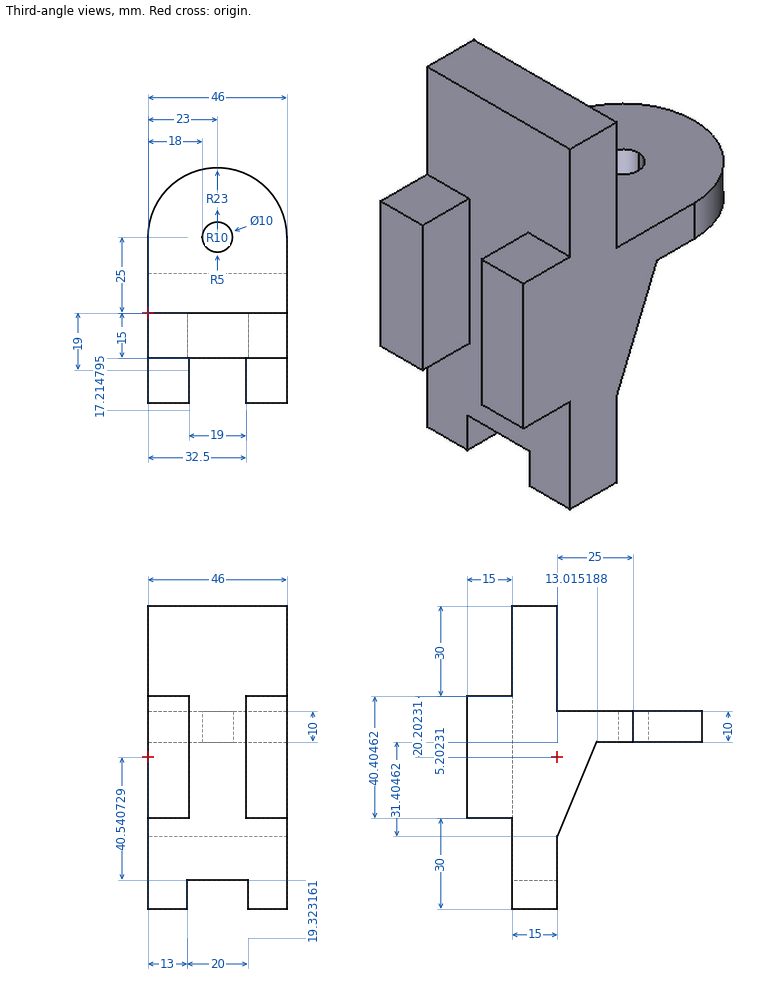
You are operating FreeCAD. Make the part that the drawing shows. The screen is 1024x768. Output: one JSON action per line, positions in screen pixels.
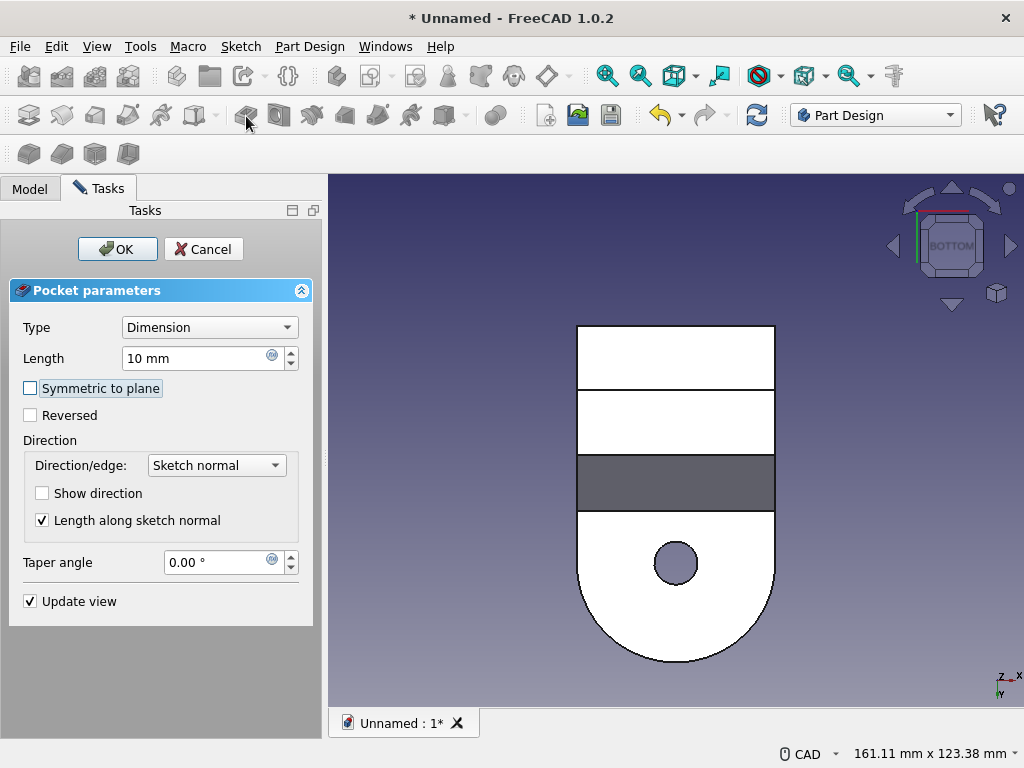
{"action": "left_click", "coordinate": [118, 249]}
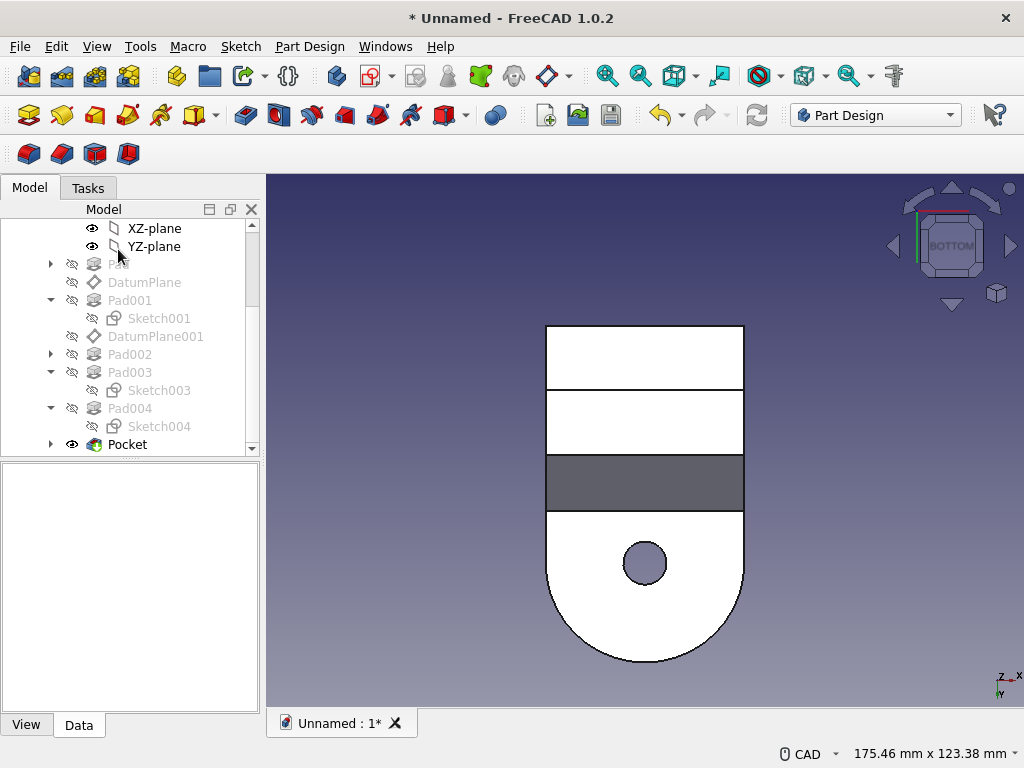
{"action": "left_click", "coordinate": [370, 76]}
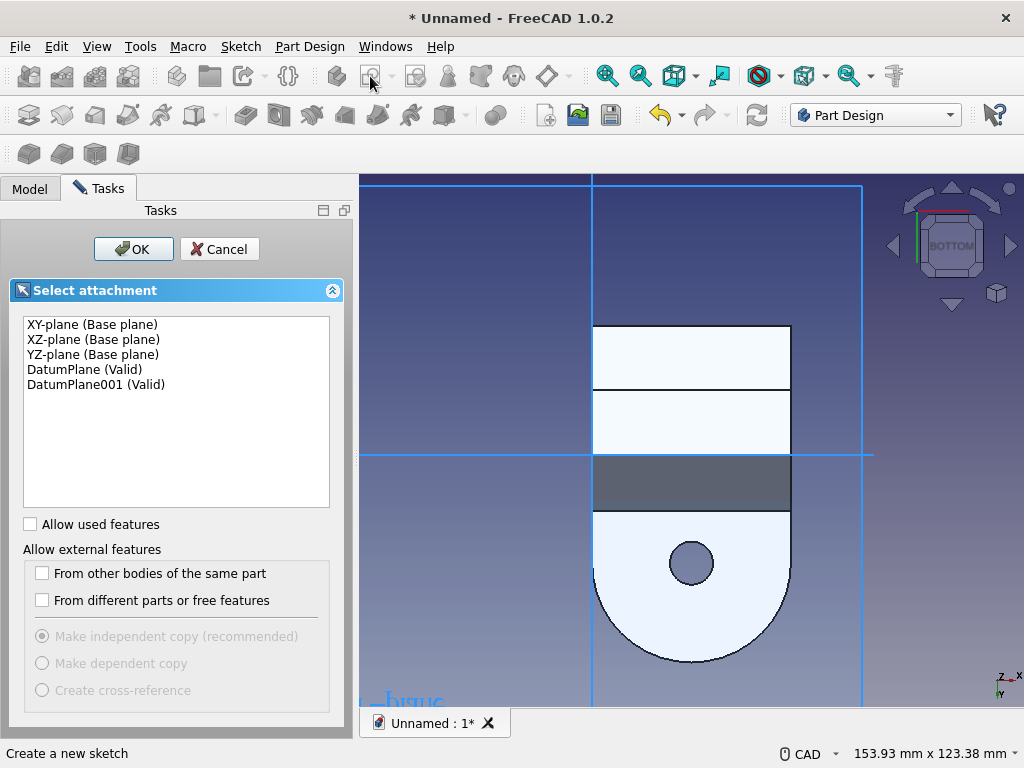
{"action": "left_click", "coordinate": [84, 340]}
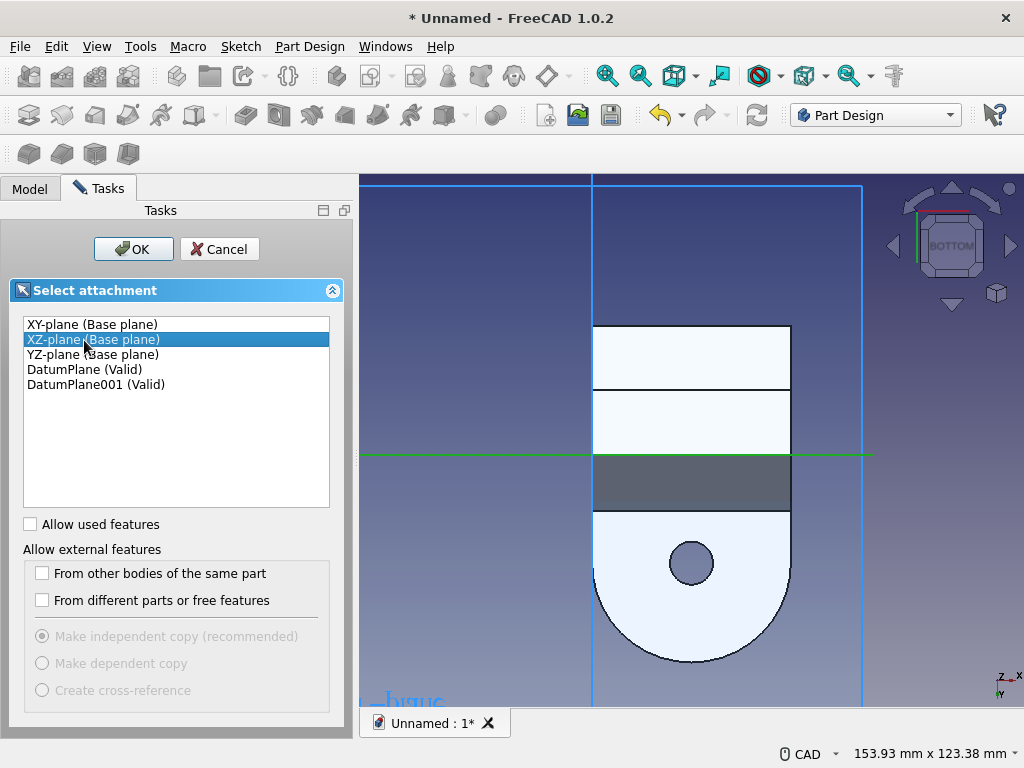
{"action": "left_click", "coordinate": [134, 249]}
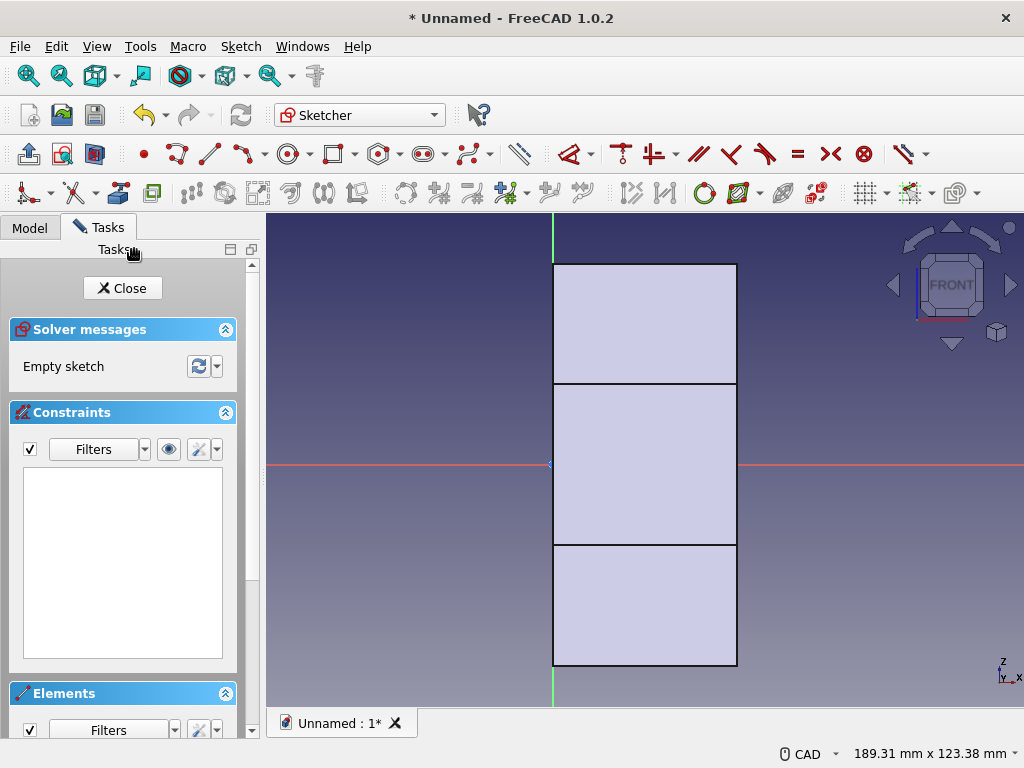
{"action": "key", "text": "q s"}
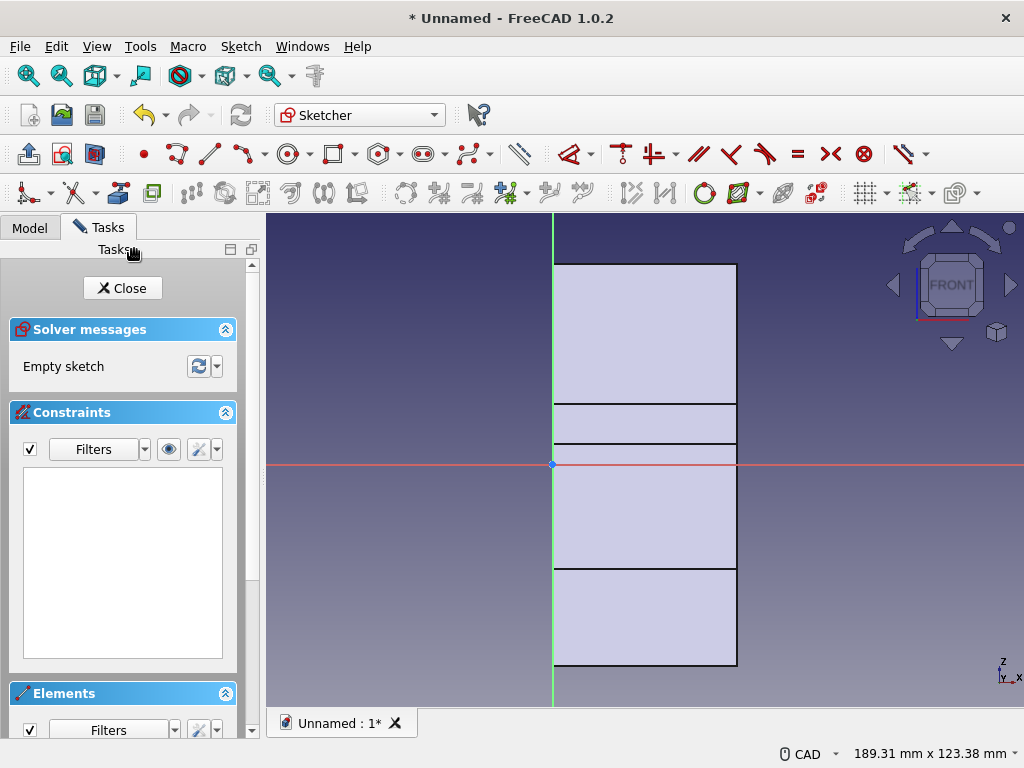
{"action": "scroll", "coordinate": [576, 460], "scroll_direction": "down", "scroll_amount": 5}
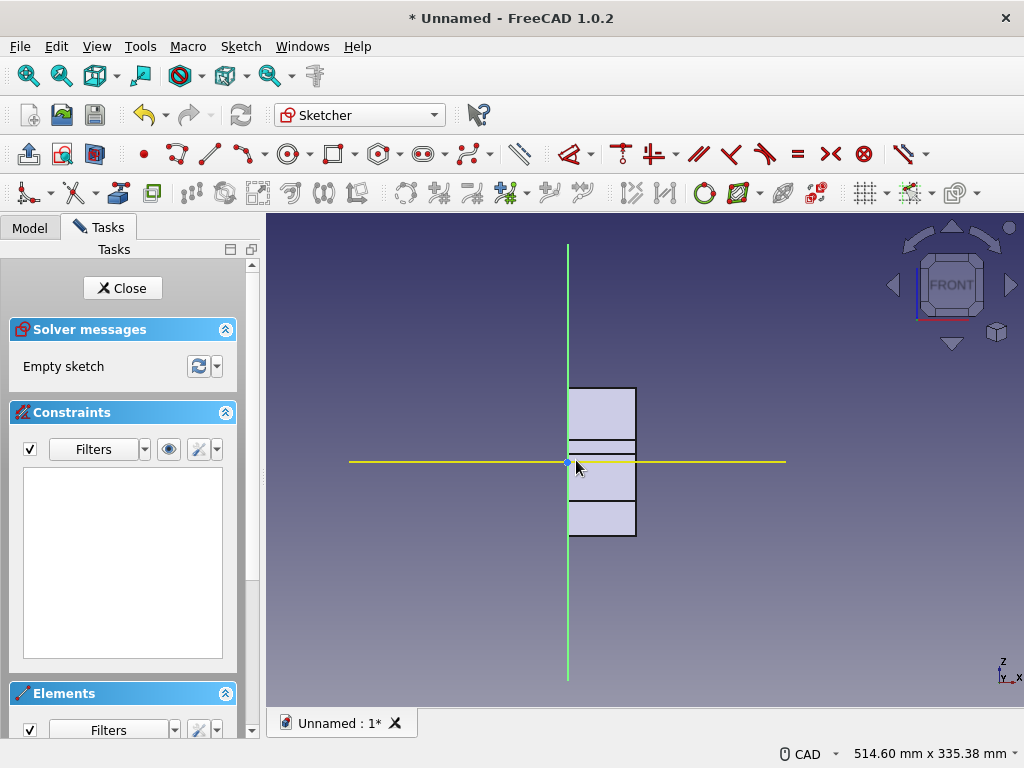
{"action": "scroll", "coordinate": [604, 544], "scroll_direction": "up", "scroll_amount": 12}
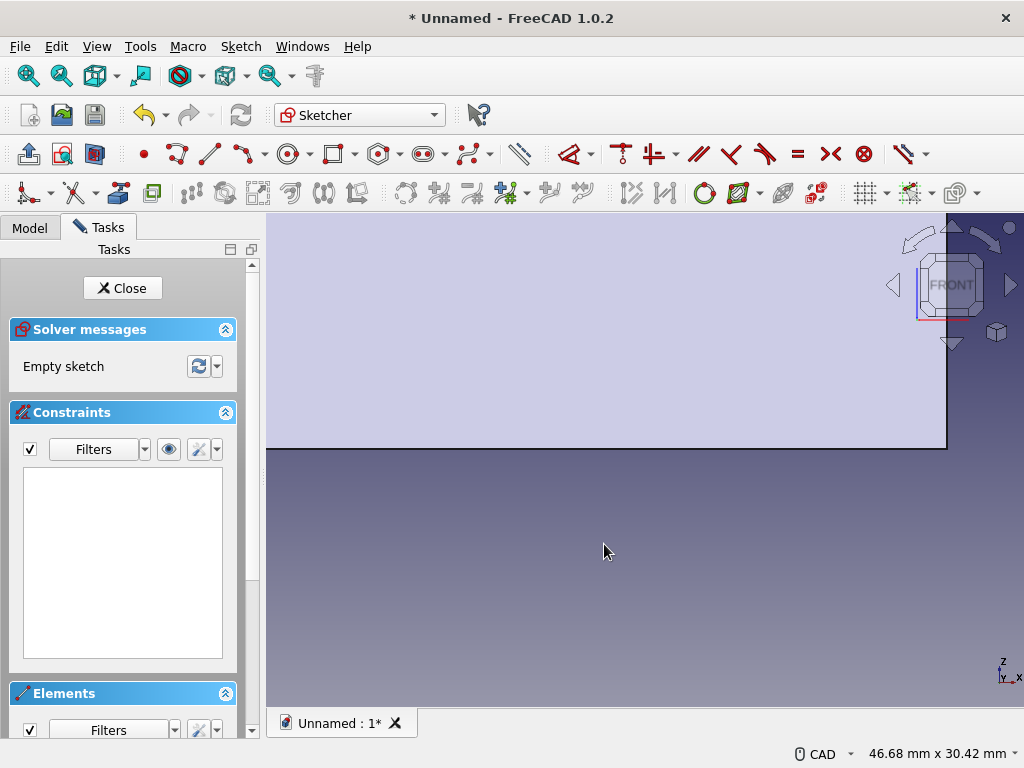
{"action": "left_click", "coordinate": [332, 154]}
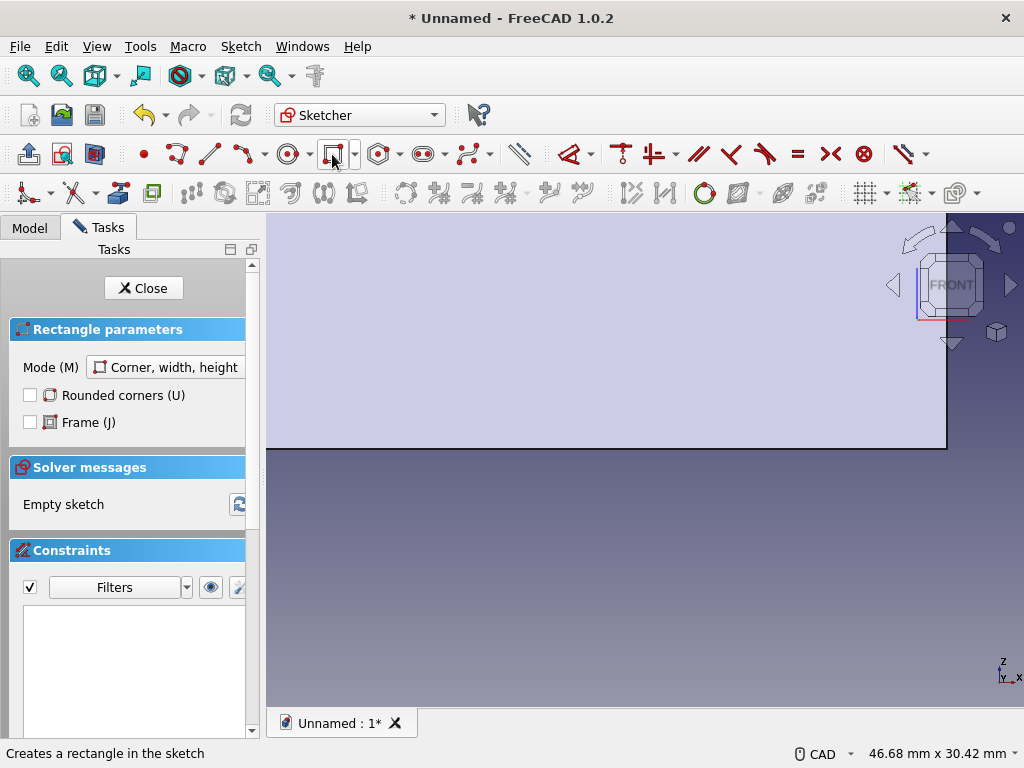
{"action": "left_click", "coordinate": [411, 292]}
{"action": "mouse_move", "coordinate": [736, 605]}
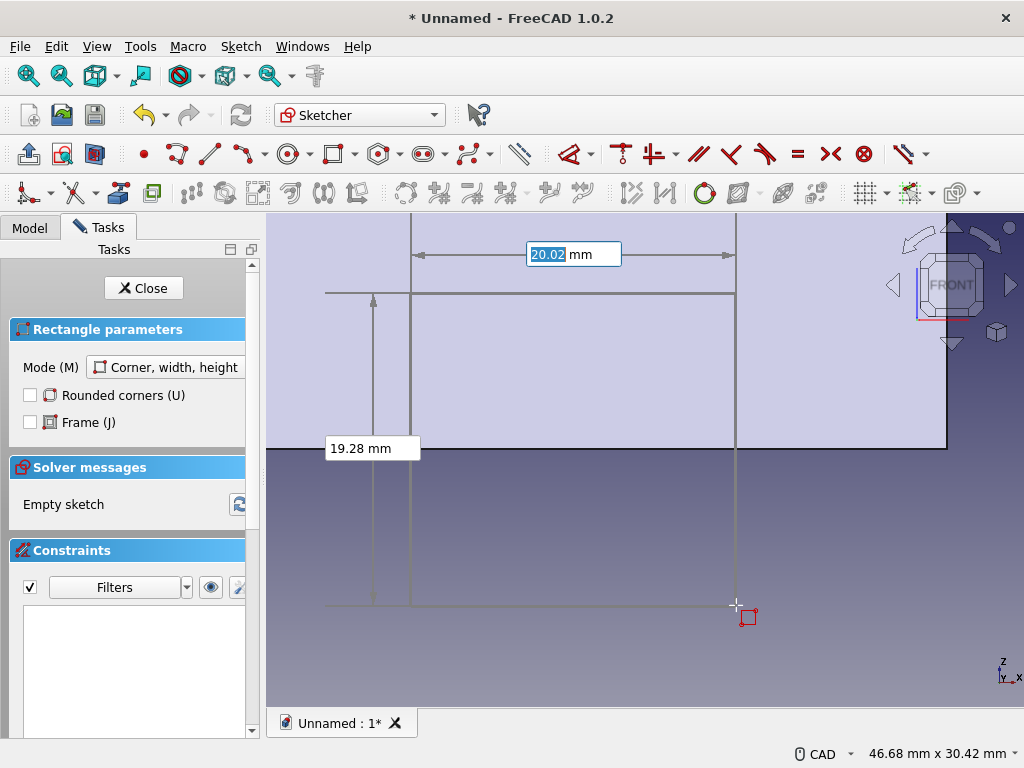
{"action": "type", "text": "20"}
{"action": "key", "text": "Tab"}
{"action": "type", "text": "19.323161"}
{"action": "key", "text": "Return"}
{"action": "key", "text": "Escape"}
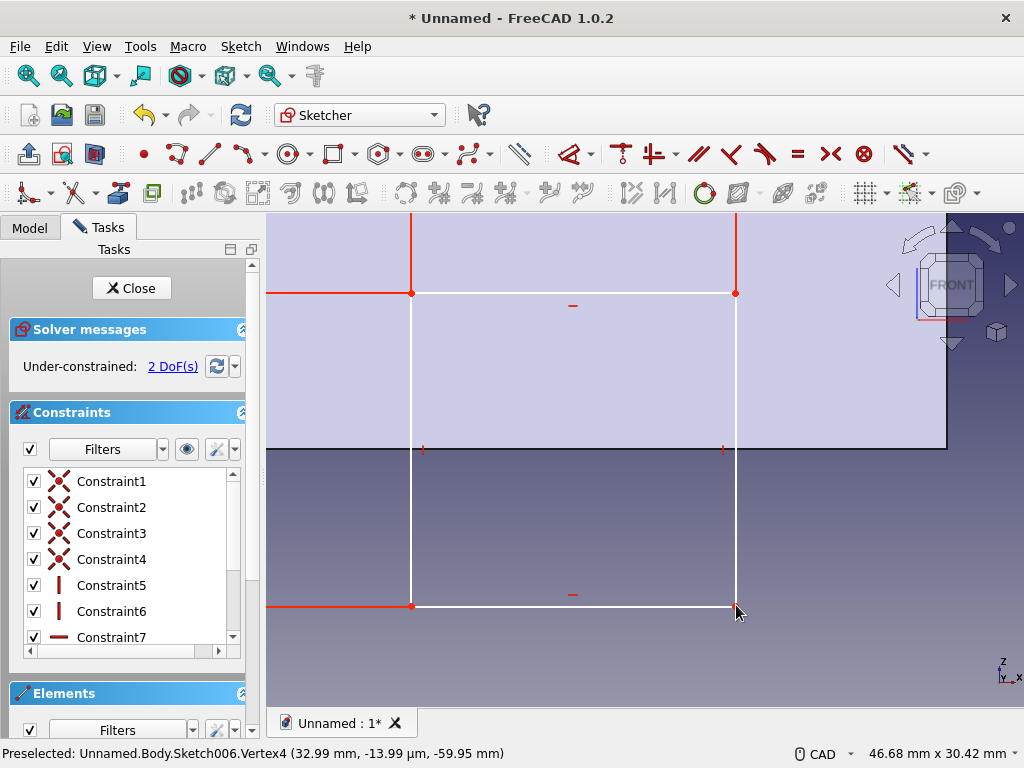
{"action": "key", "text": "d"}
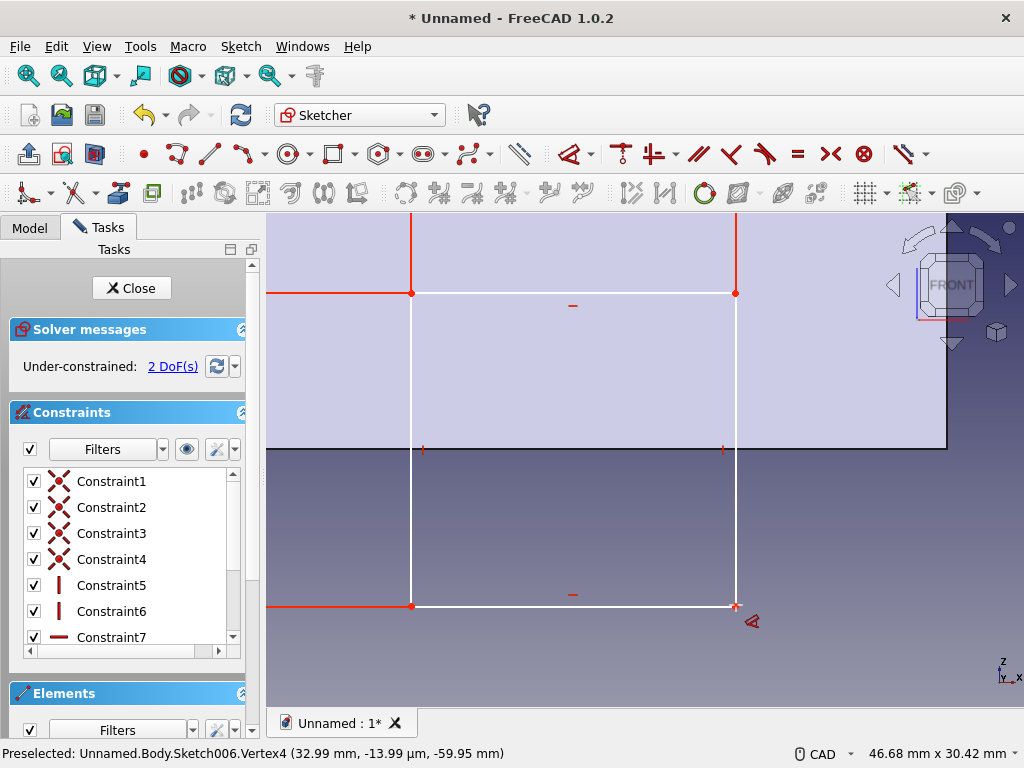
{"action": "left_click", "coordinate": [411, 293]}
{"action": "left_click", "coordinate": [352, 327]}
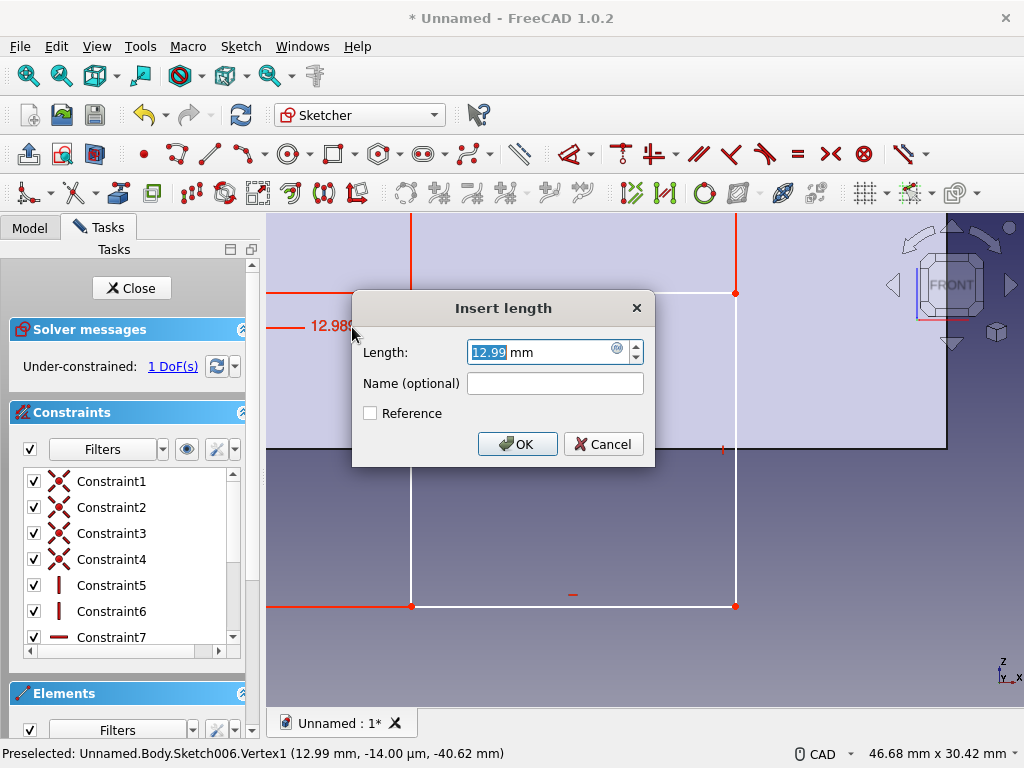
{"action": "type", "text": "13"}
{"action": "key", "text": "Return"}